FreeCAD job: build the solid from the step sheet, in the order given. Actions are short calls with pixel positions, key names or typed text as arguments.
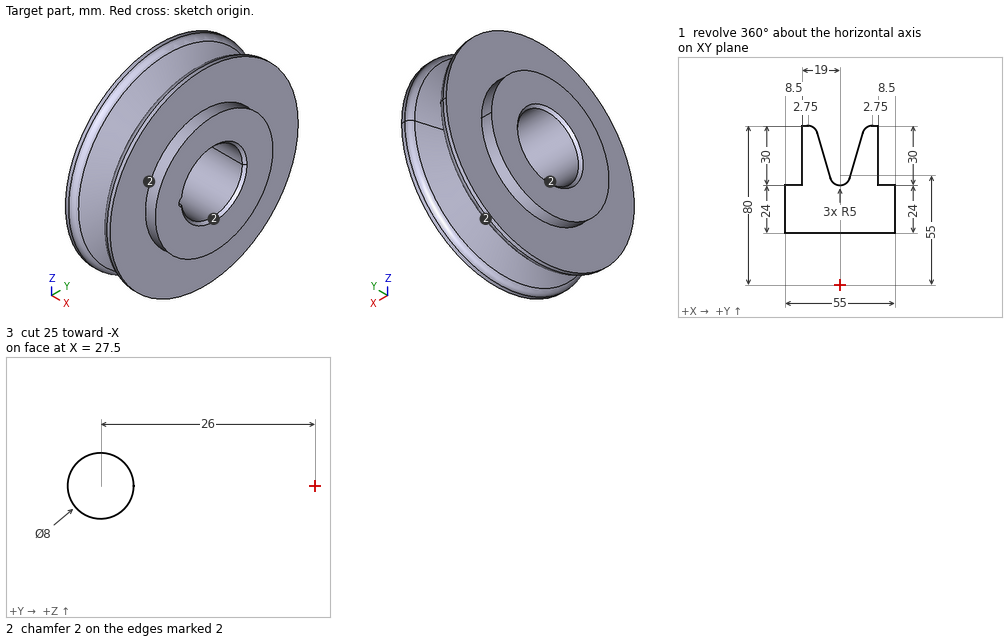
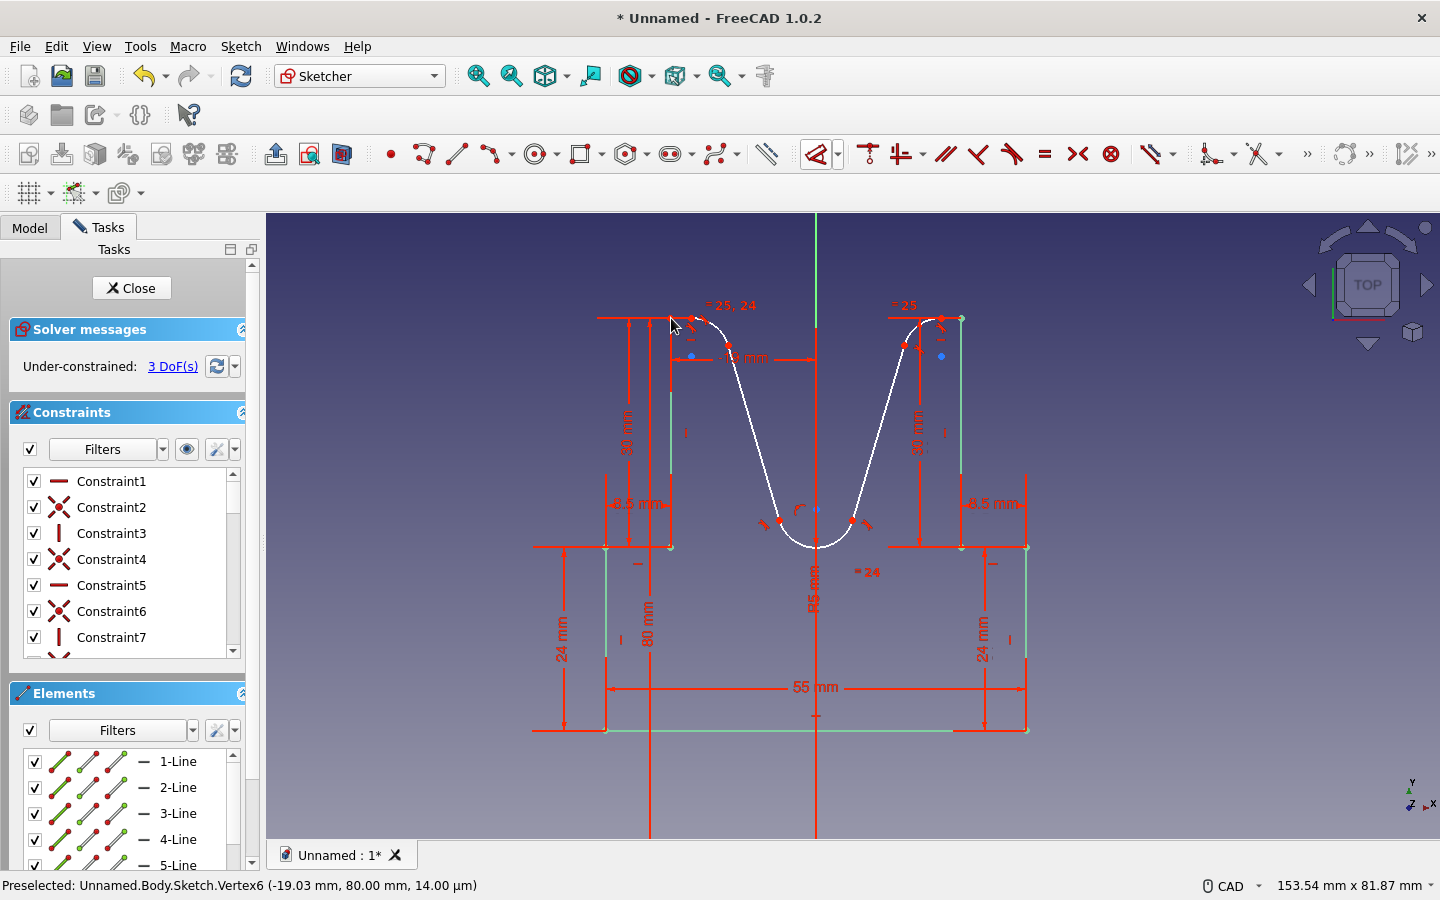
click(816, 509)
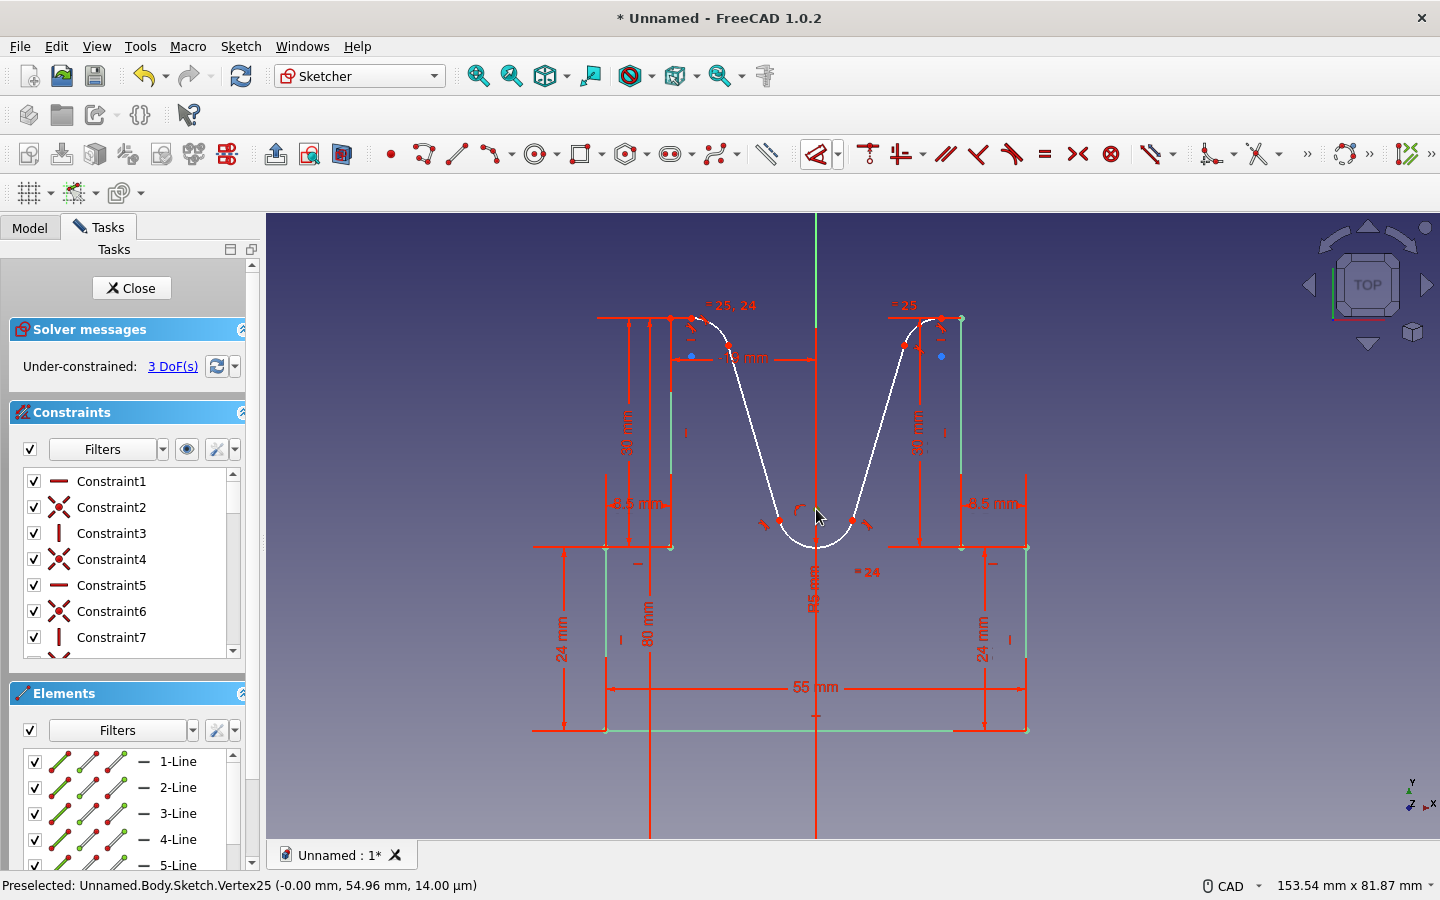
click(838, 154)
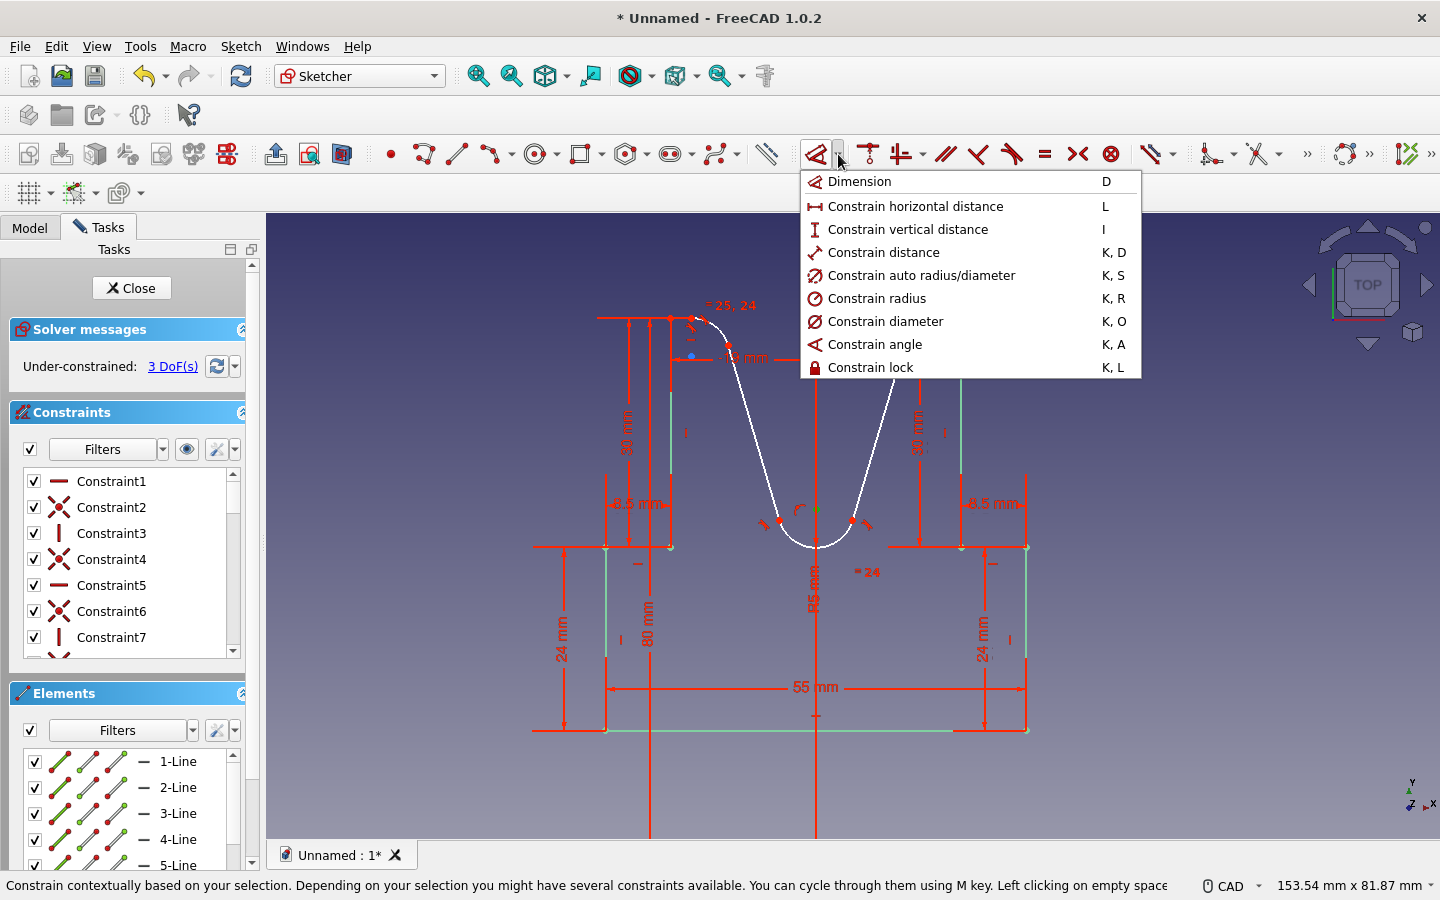
click(971, 230)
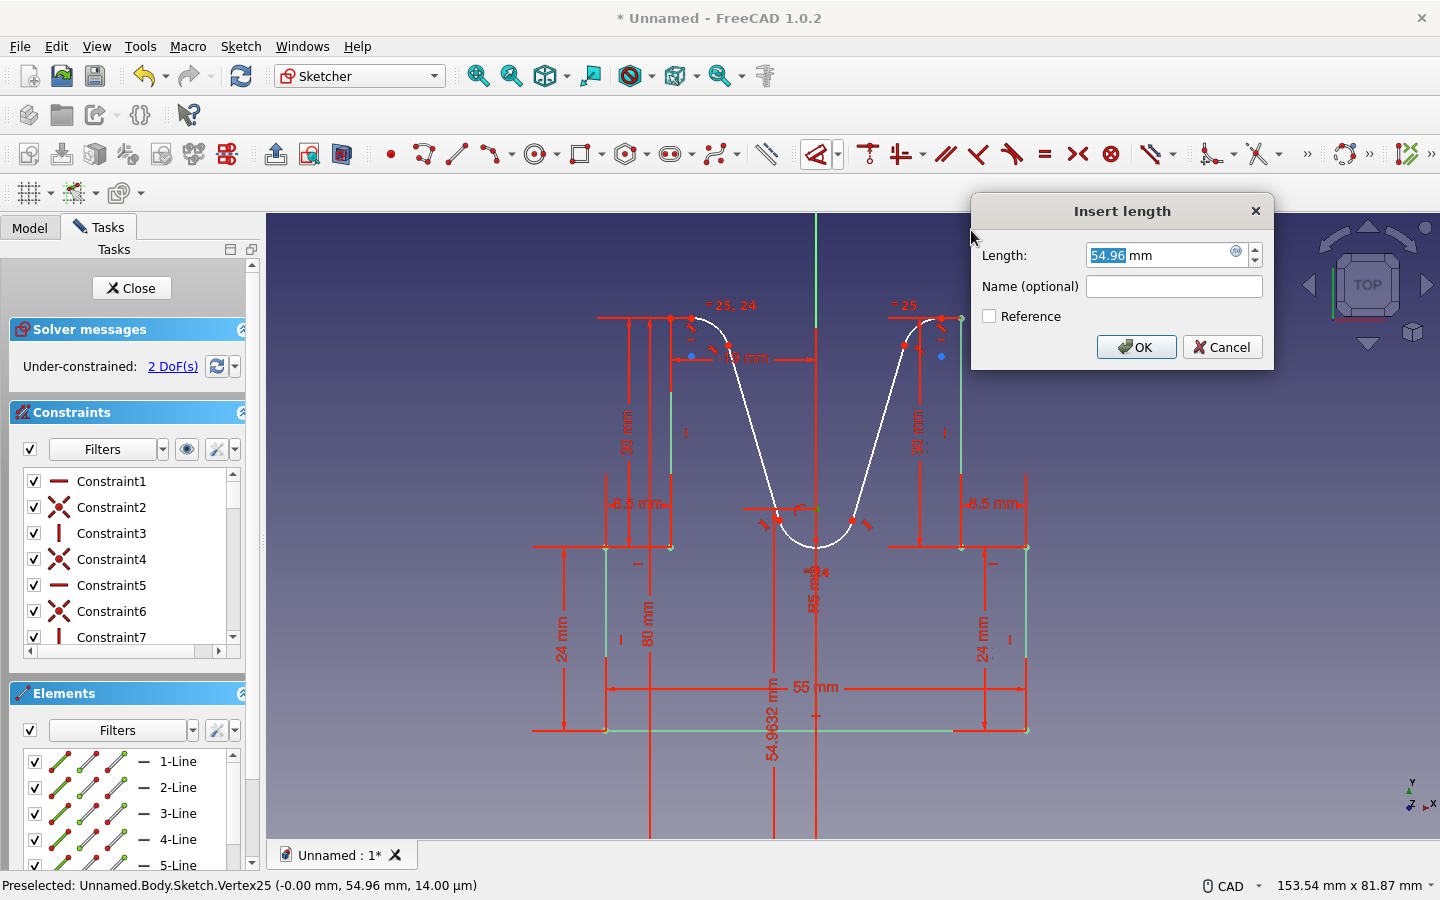
text(55)
key(Return)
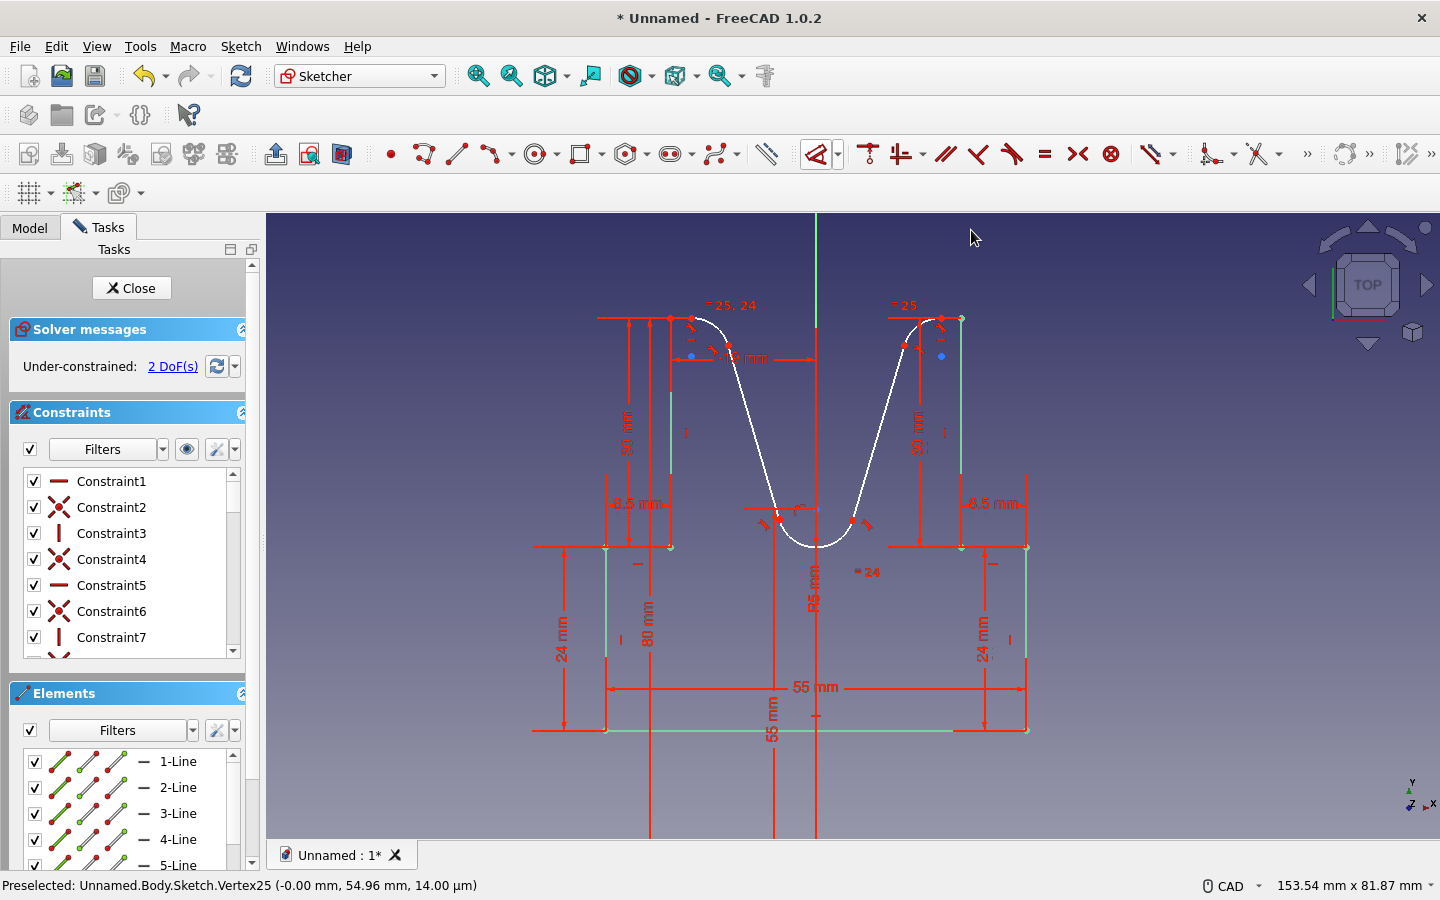
scroll(681, 318, up, 4)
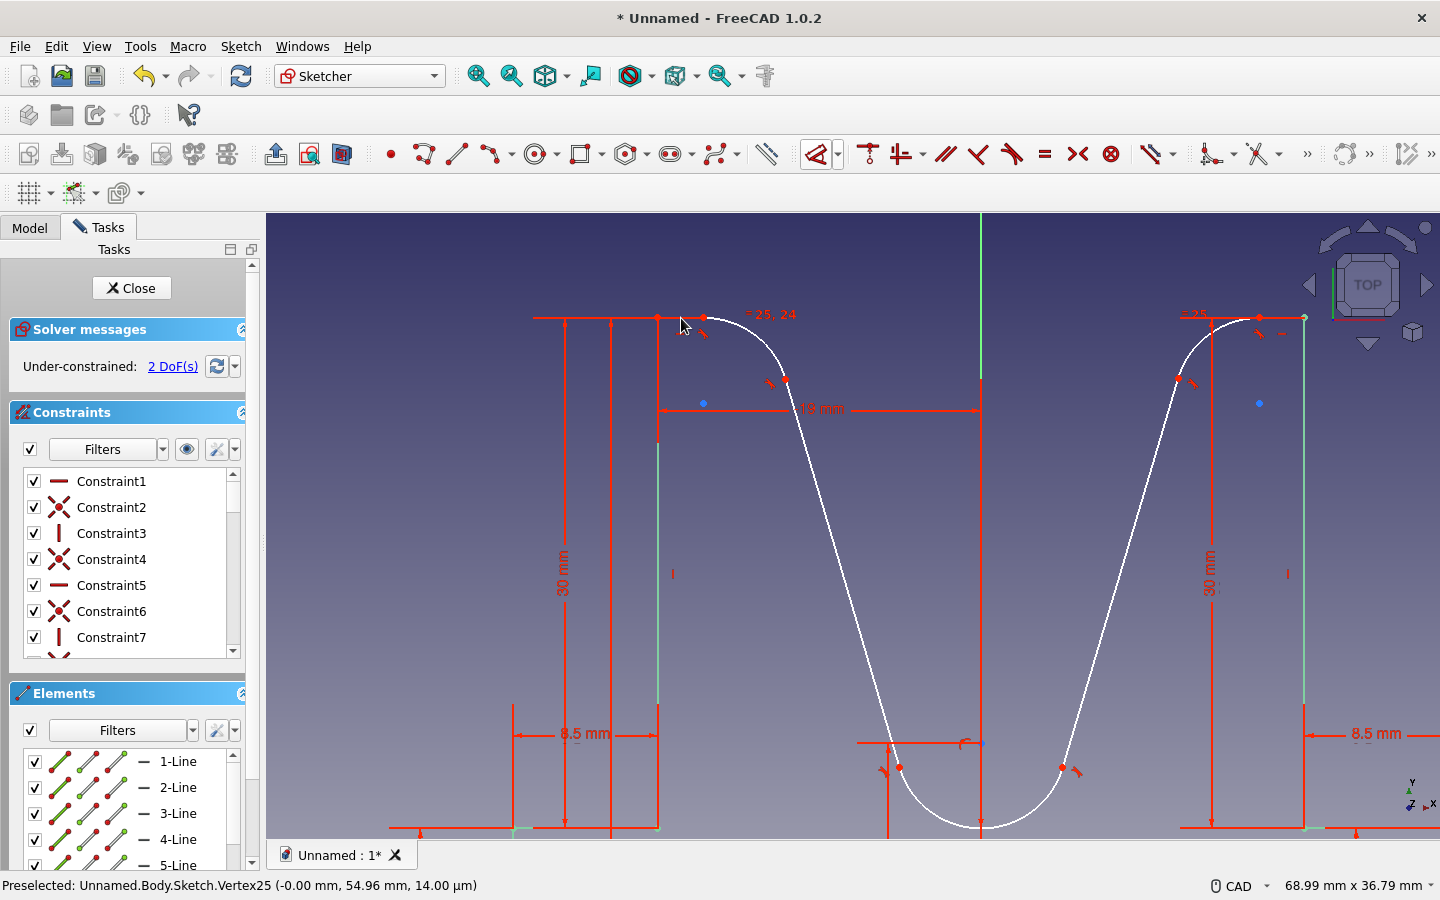
click(681, 318)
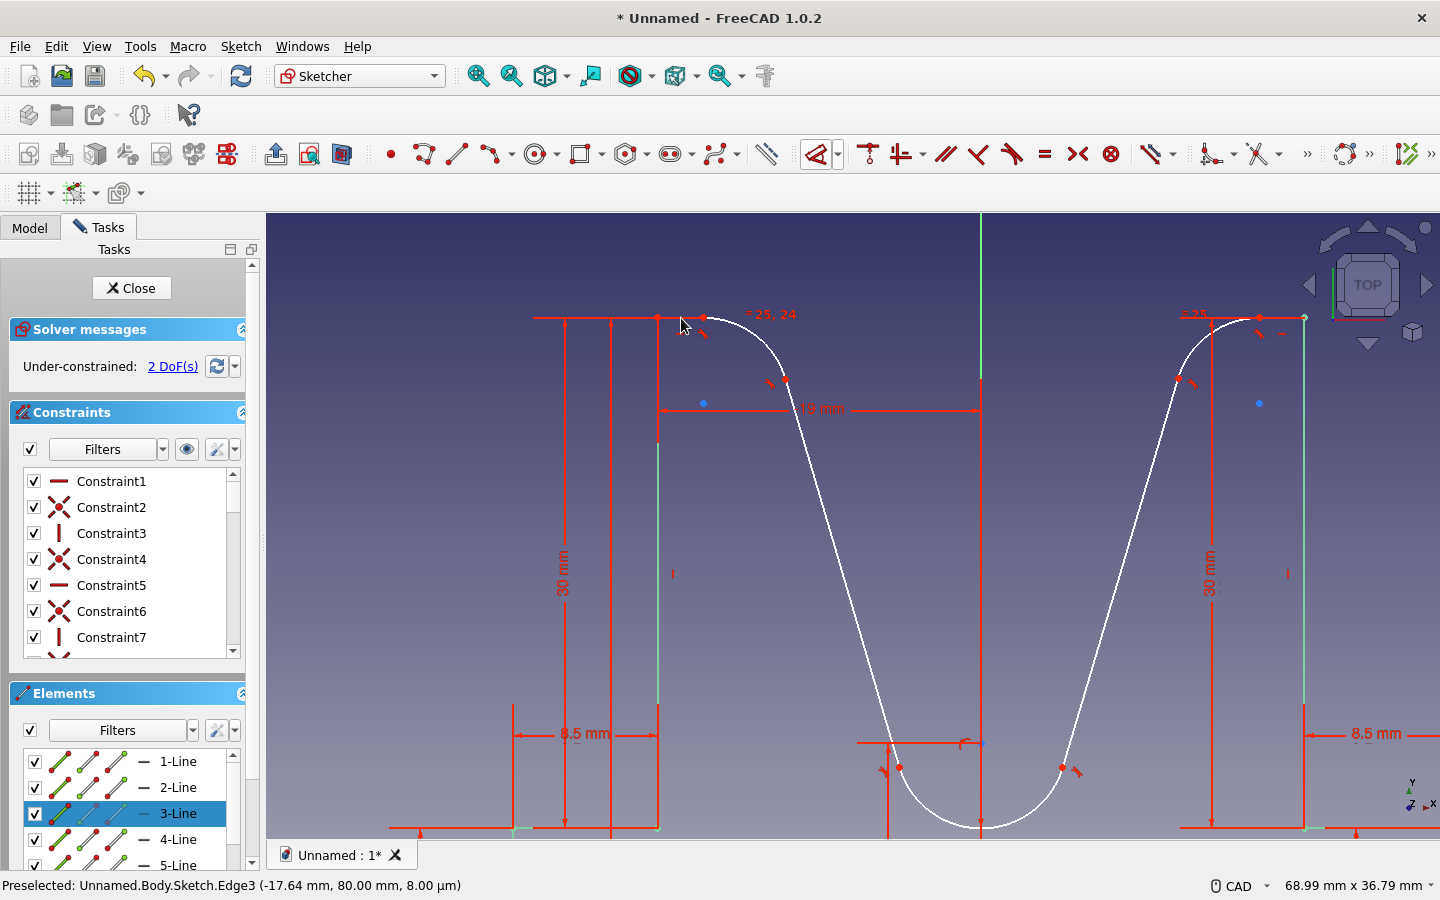
key(l)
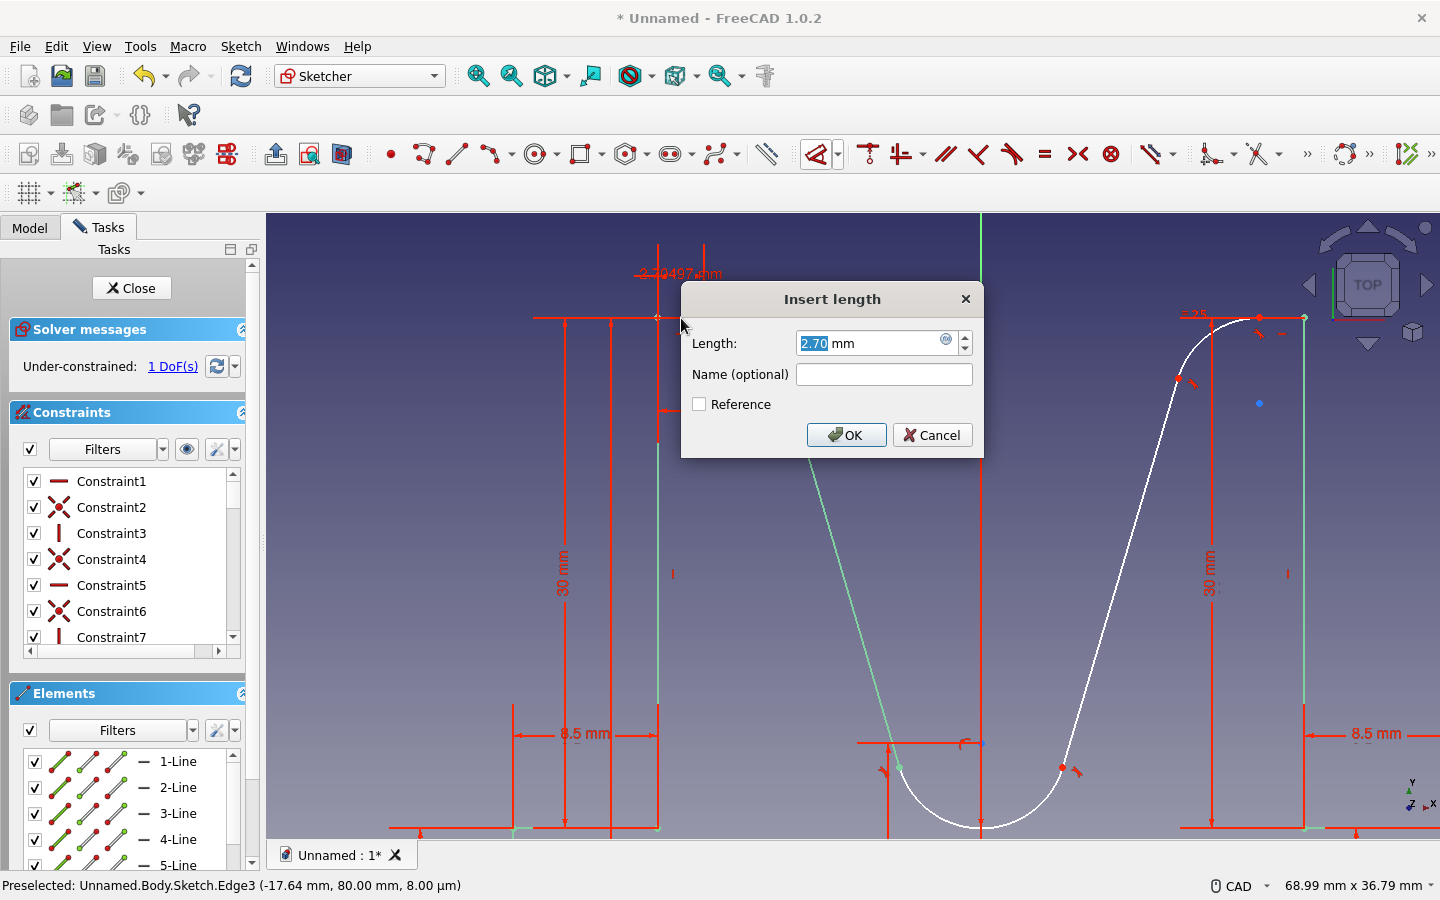
text(2.75)
key(Return)